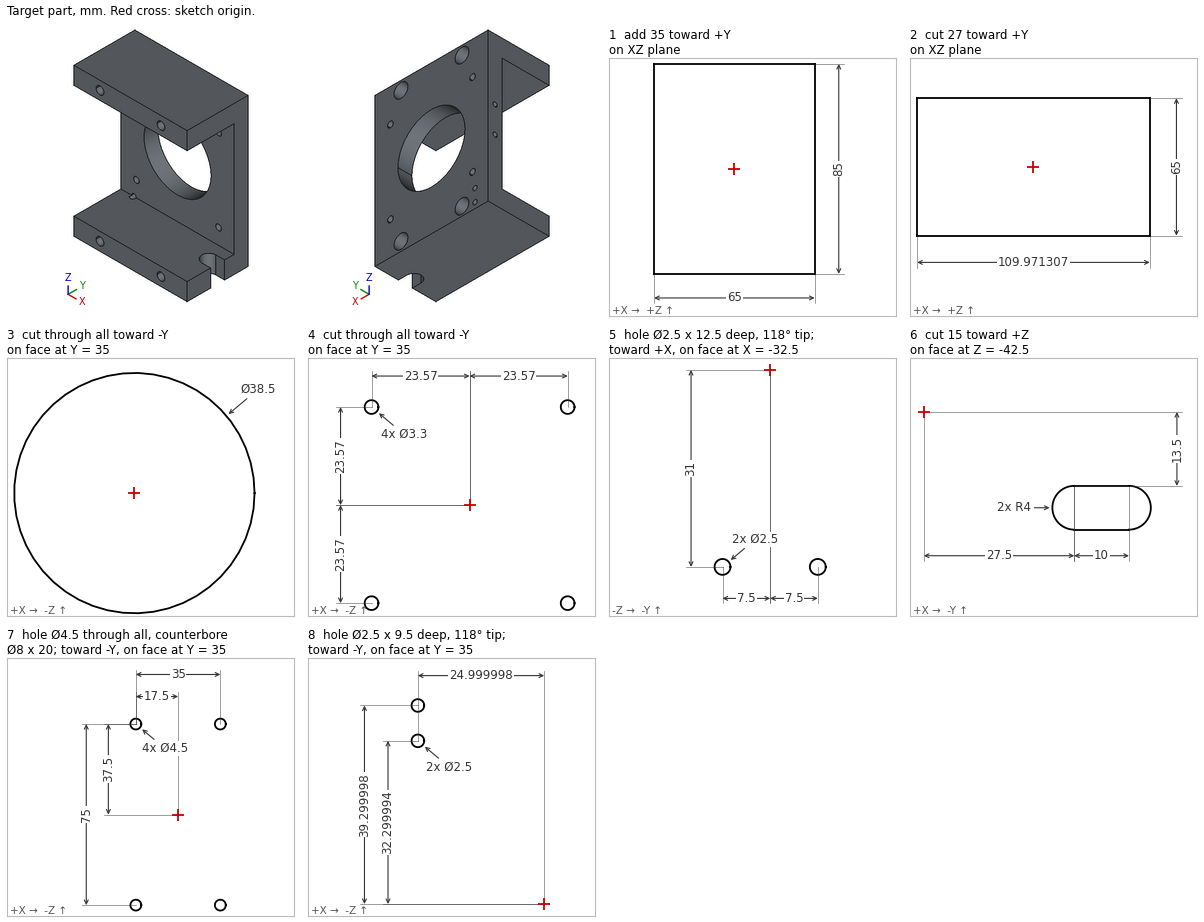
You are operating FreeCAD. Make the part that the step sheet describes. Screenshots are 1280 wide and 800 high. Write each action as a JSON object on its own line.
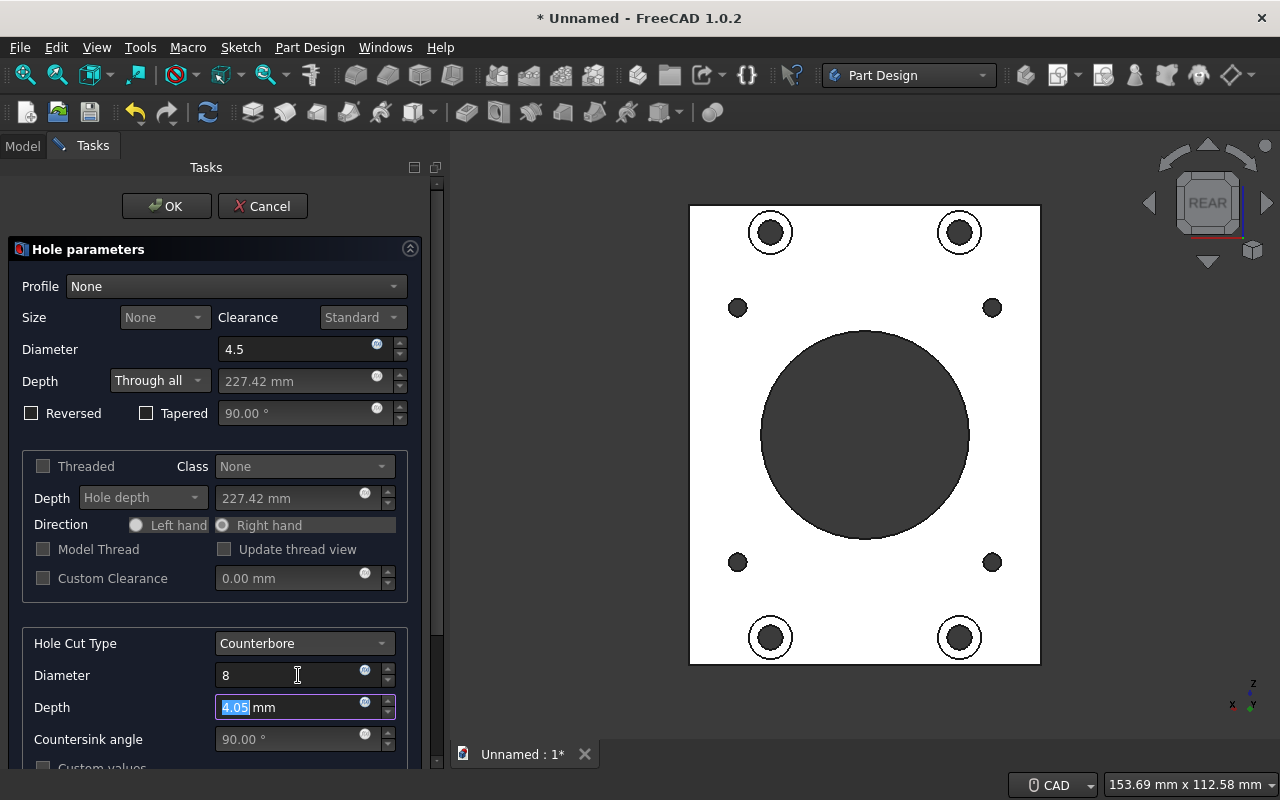
{"action": "type", "text": "20"}
{"action": "key", "text": "Tab"}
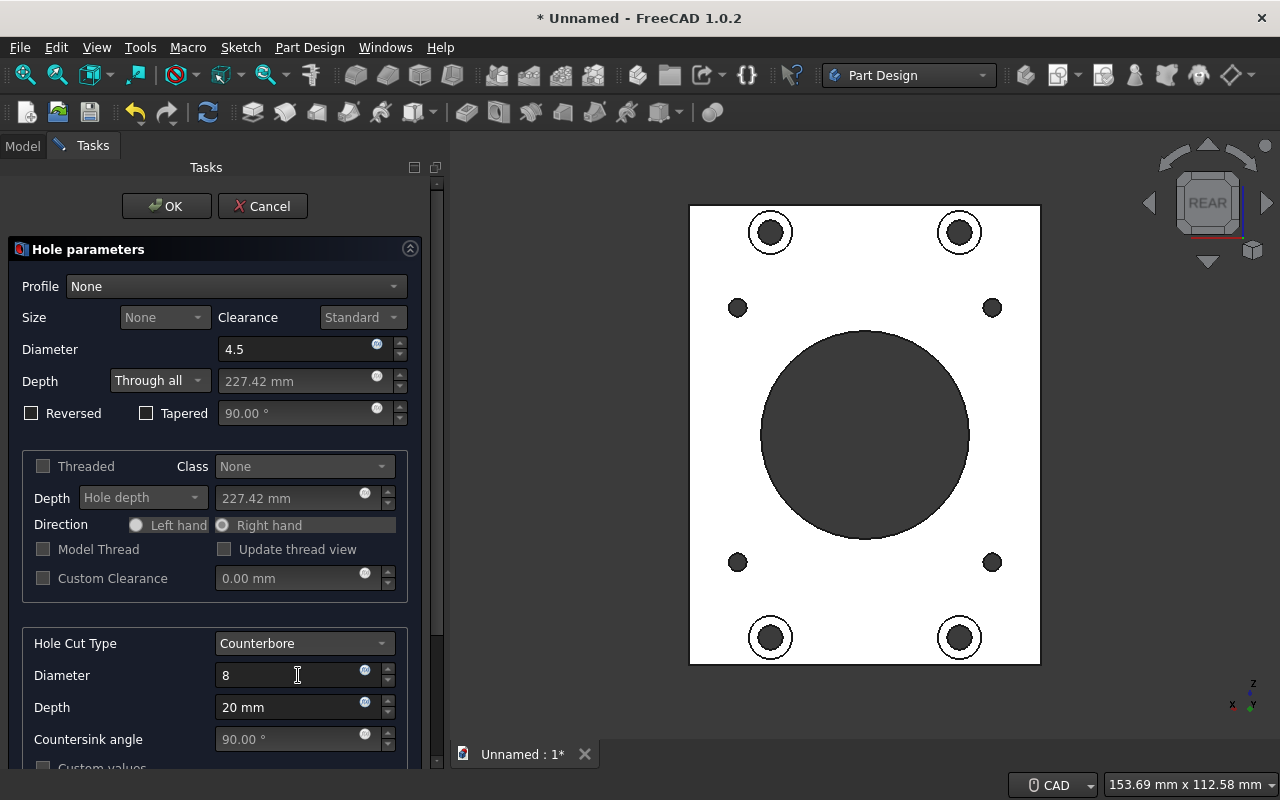
{"action": "left_click", "coordinate": [167, 206]}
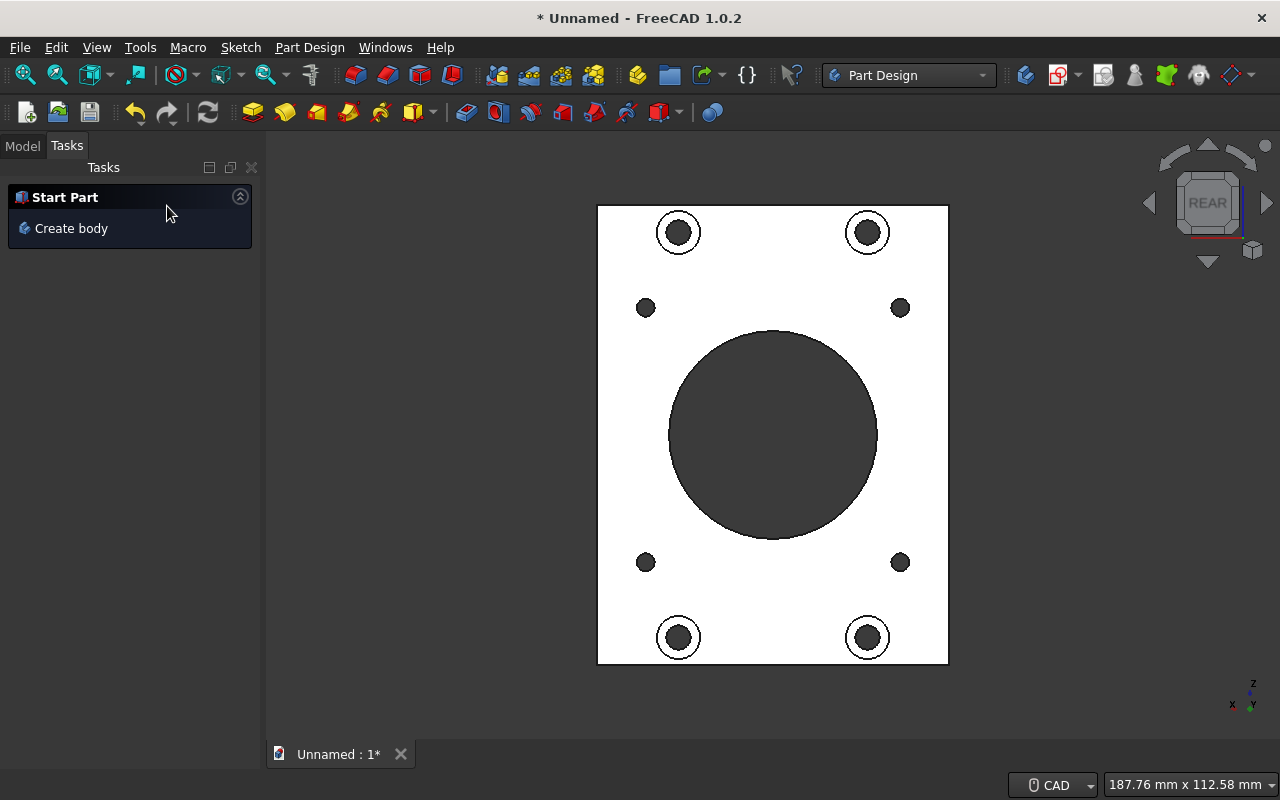
{"action": "left_click", "coordinate": [723, 565]}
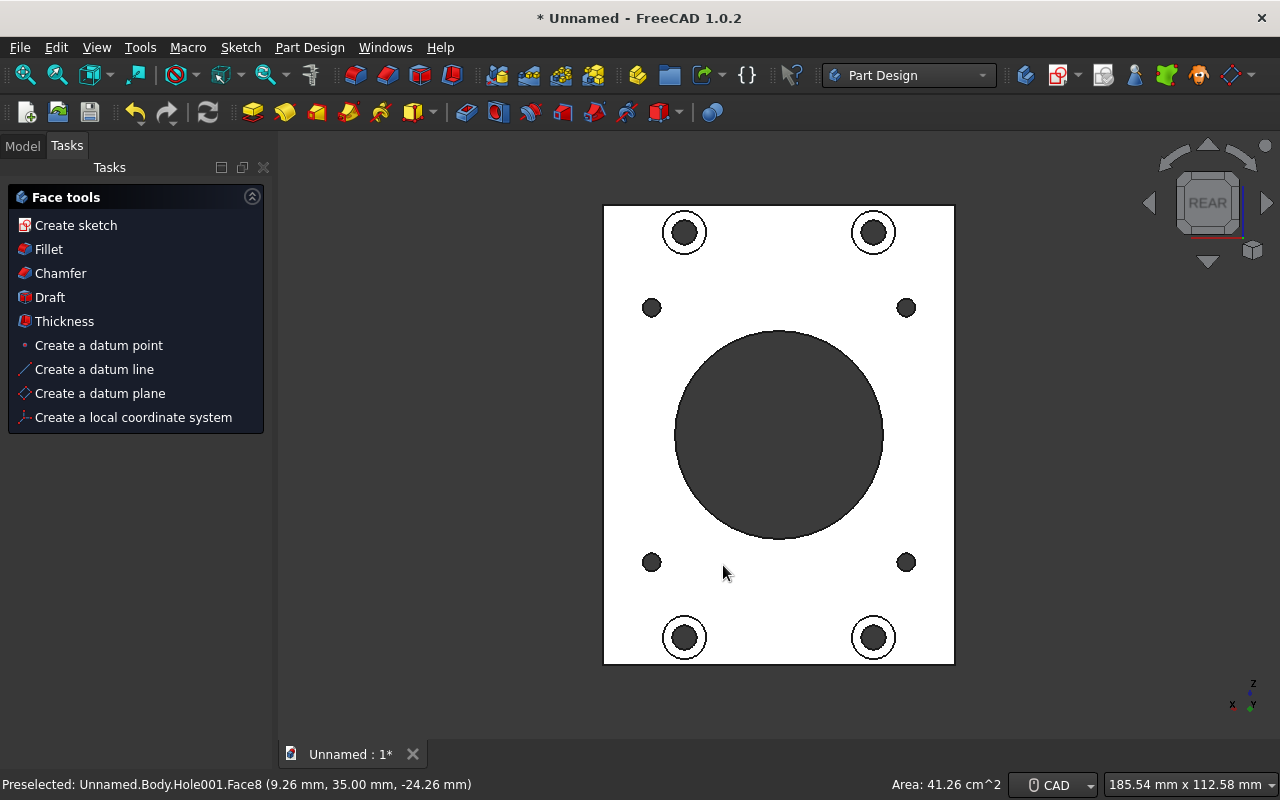
{"action": "left_click", "coordinate": [1058, 76]}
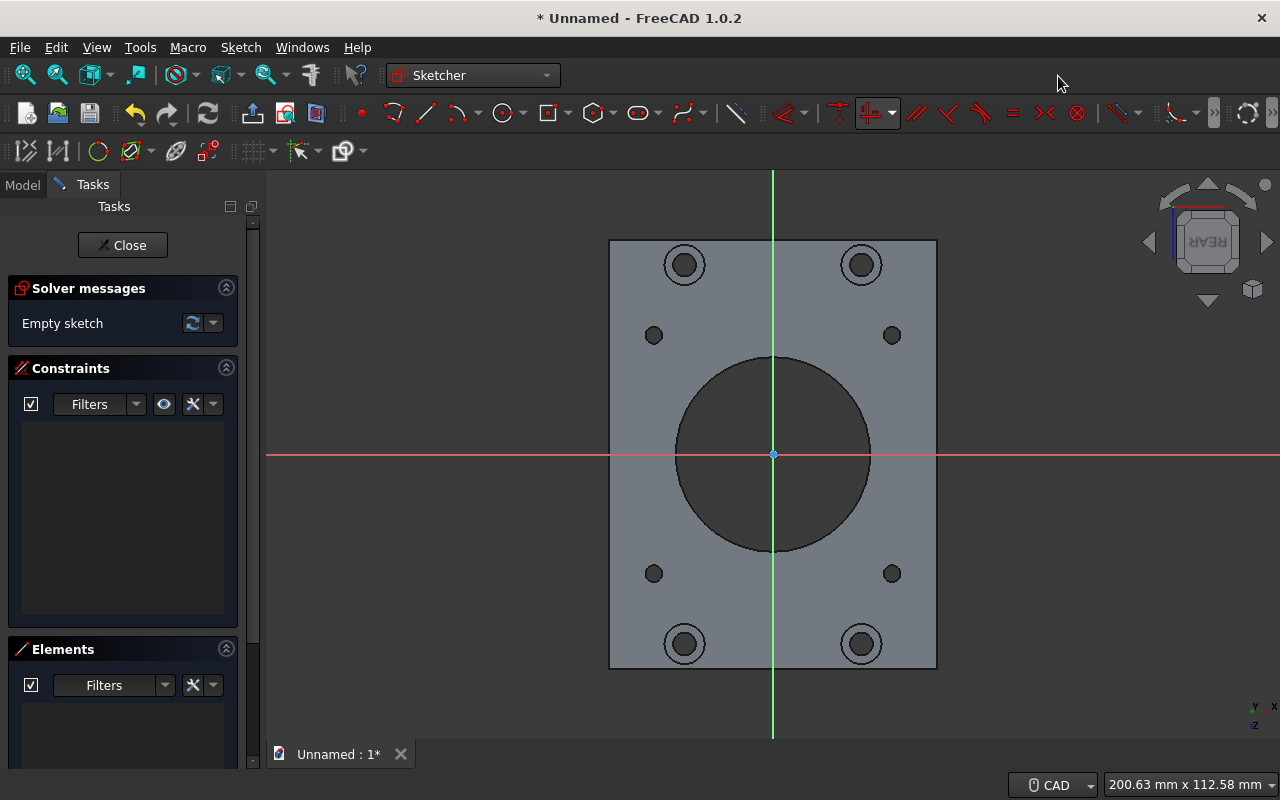
{"action": "scroll", "coordinate": [638, 245], "scroll_direction": "up", "scroll_amount": 10}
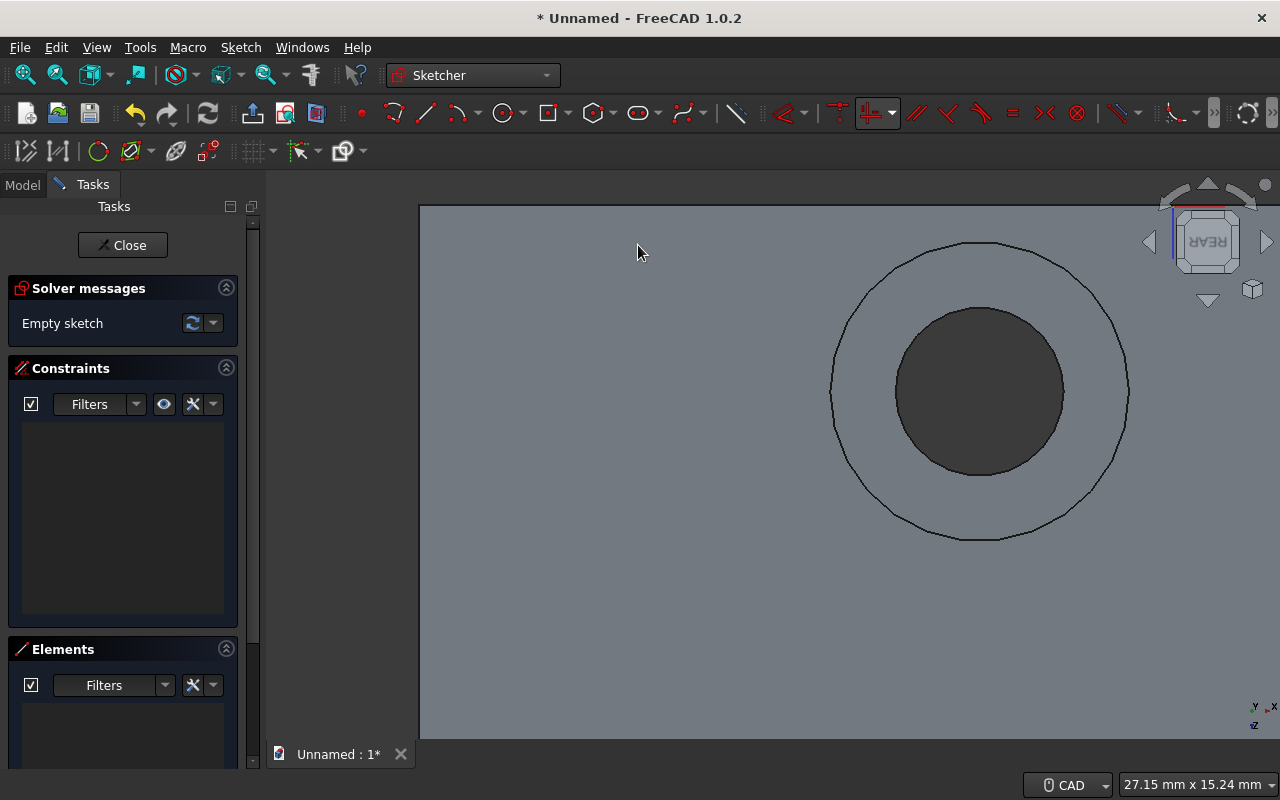
{"action": "left_click", "coordinate": [504, 114]}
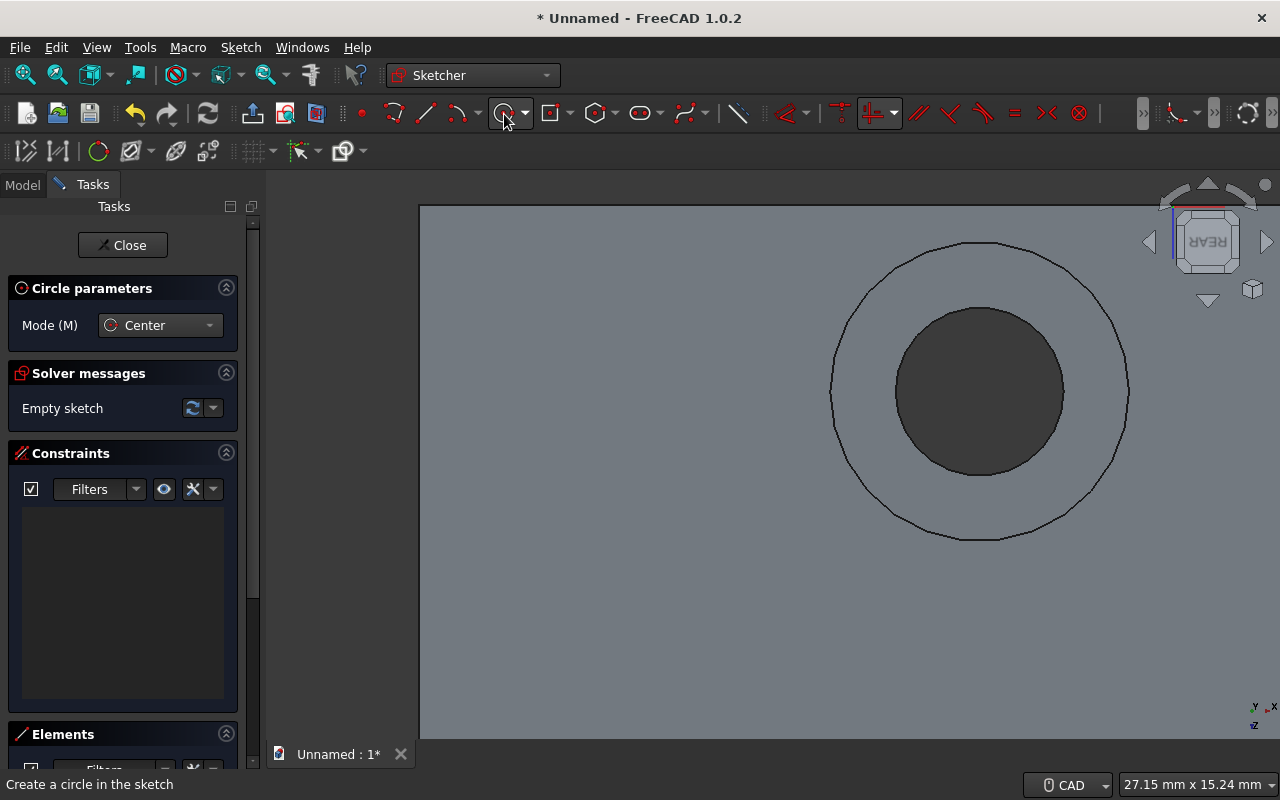
{"action": "left_click", "coordinate": [700, 586]}
{"action": "mouse_move", "coordinate": [733, 553]}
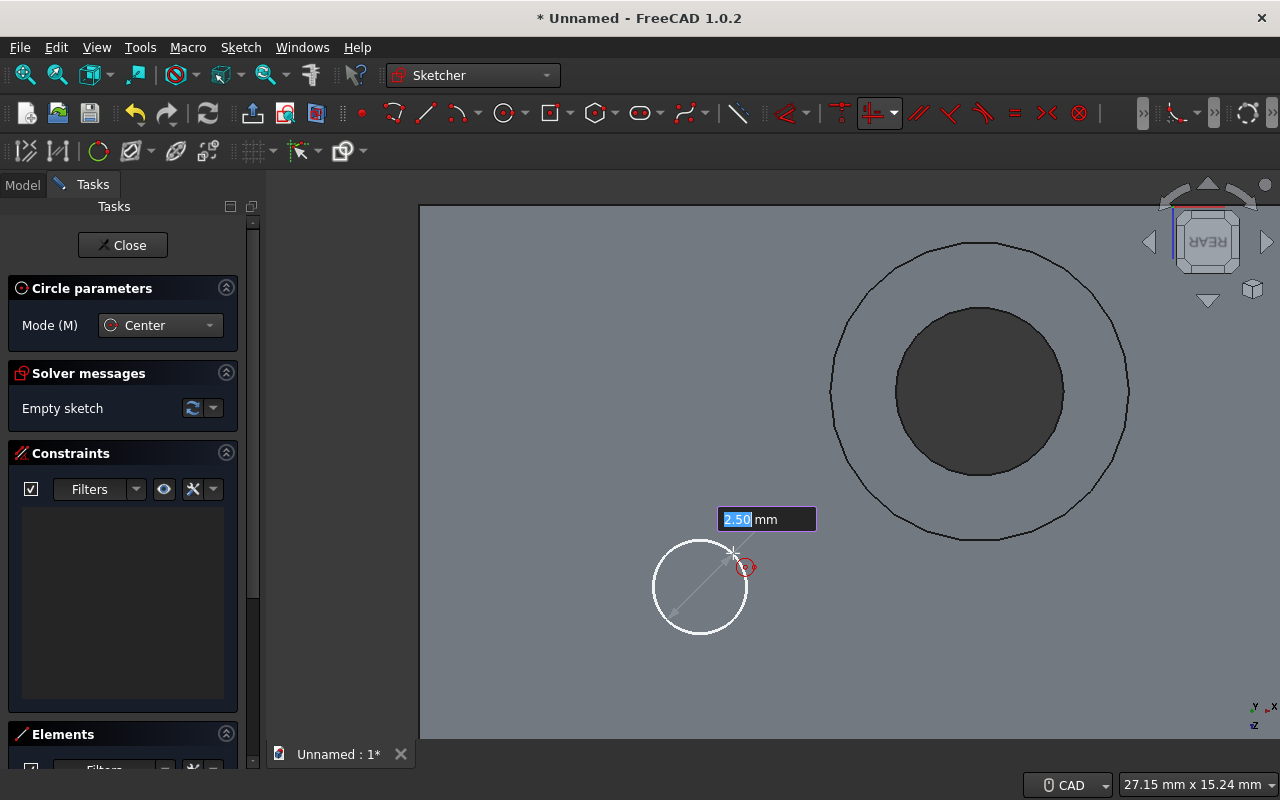
{"action": "type", "text": "2.5"}
{"action": "key", "text": "Return"}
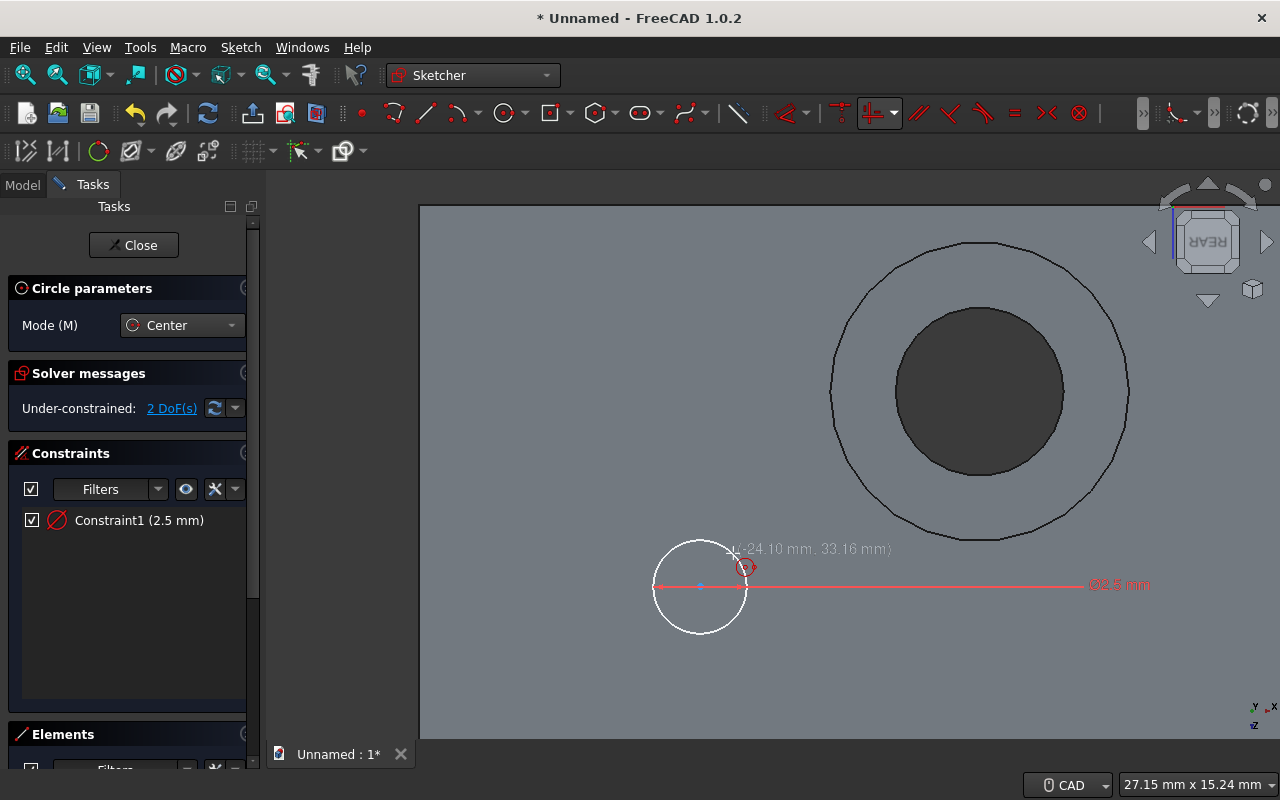
{"action": "left_click", "coordinate": [700, 325]}
{"action": "mouse_move", "coordinate": [733, 292]}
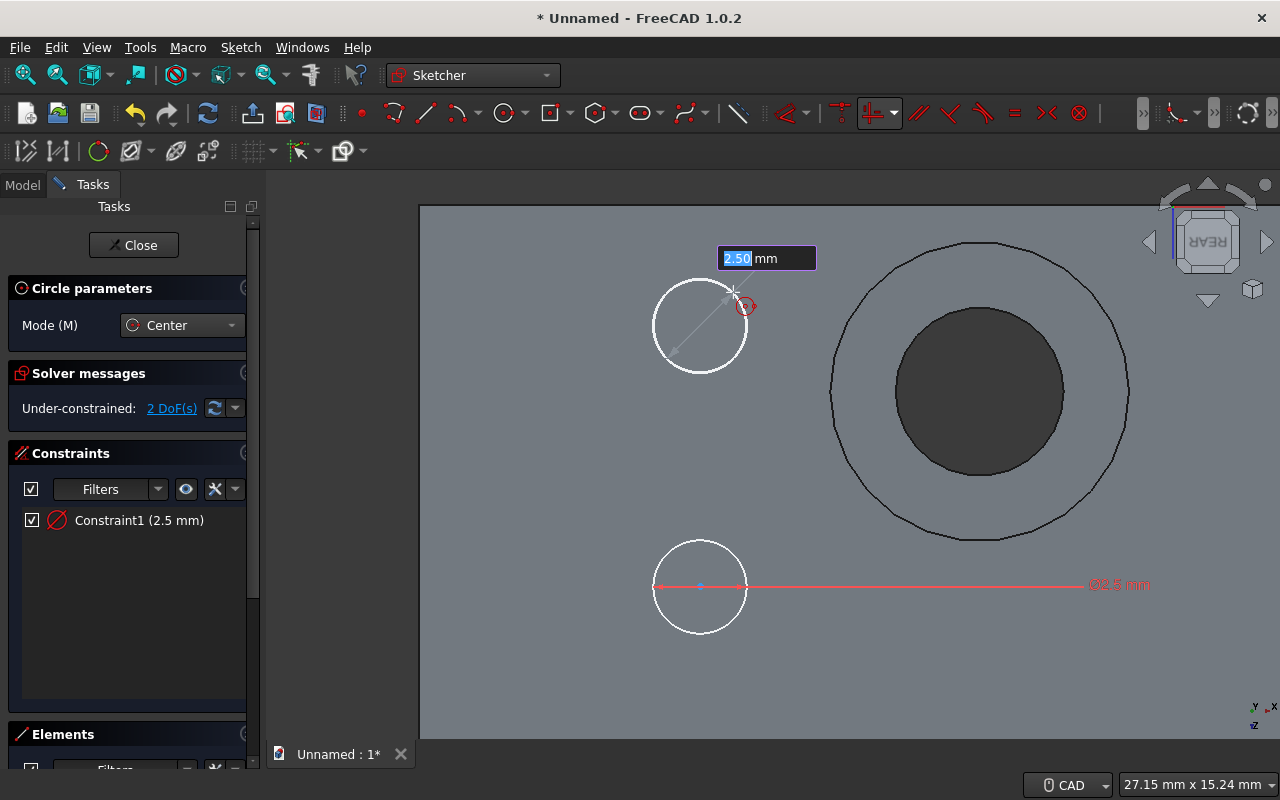
{"action": "type", "text": "2.5"}
{"action": "key", "text": "Return"}
{"action": "key", "text": "Escape"}